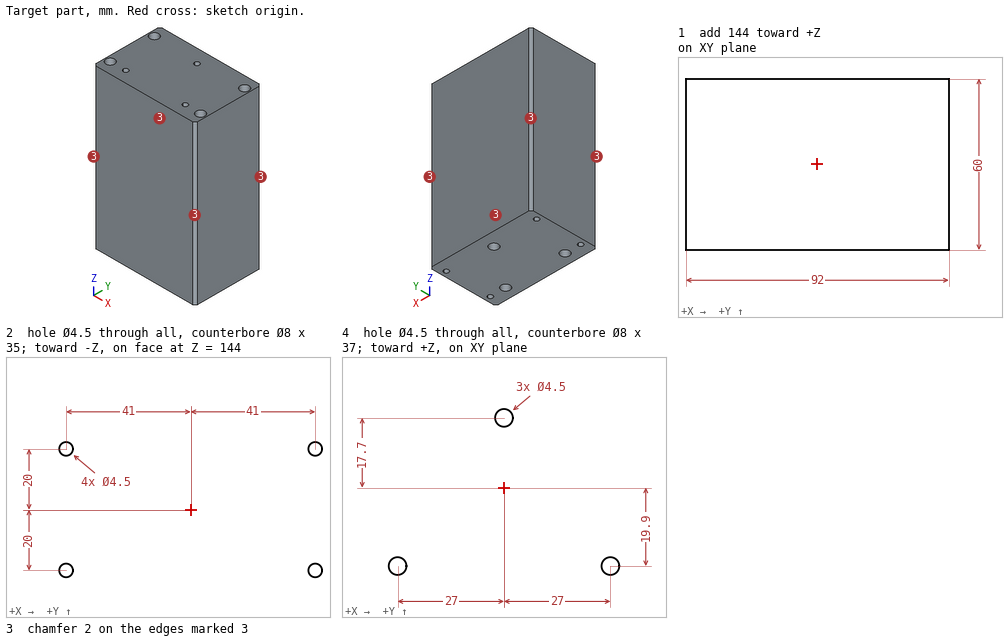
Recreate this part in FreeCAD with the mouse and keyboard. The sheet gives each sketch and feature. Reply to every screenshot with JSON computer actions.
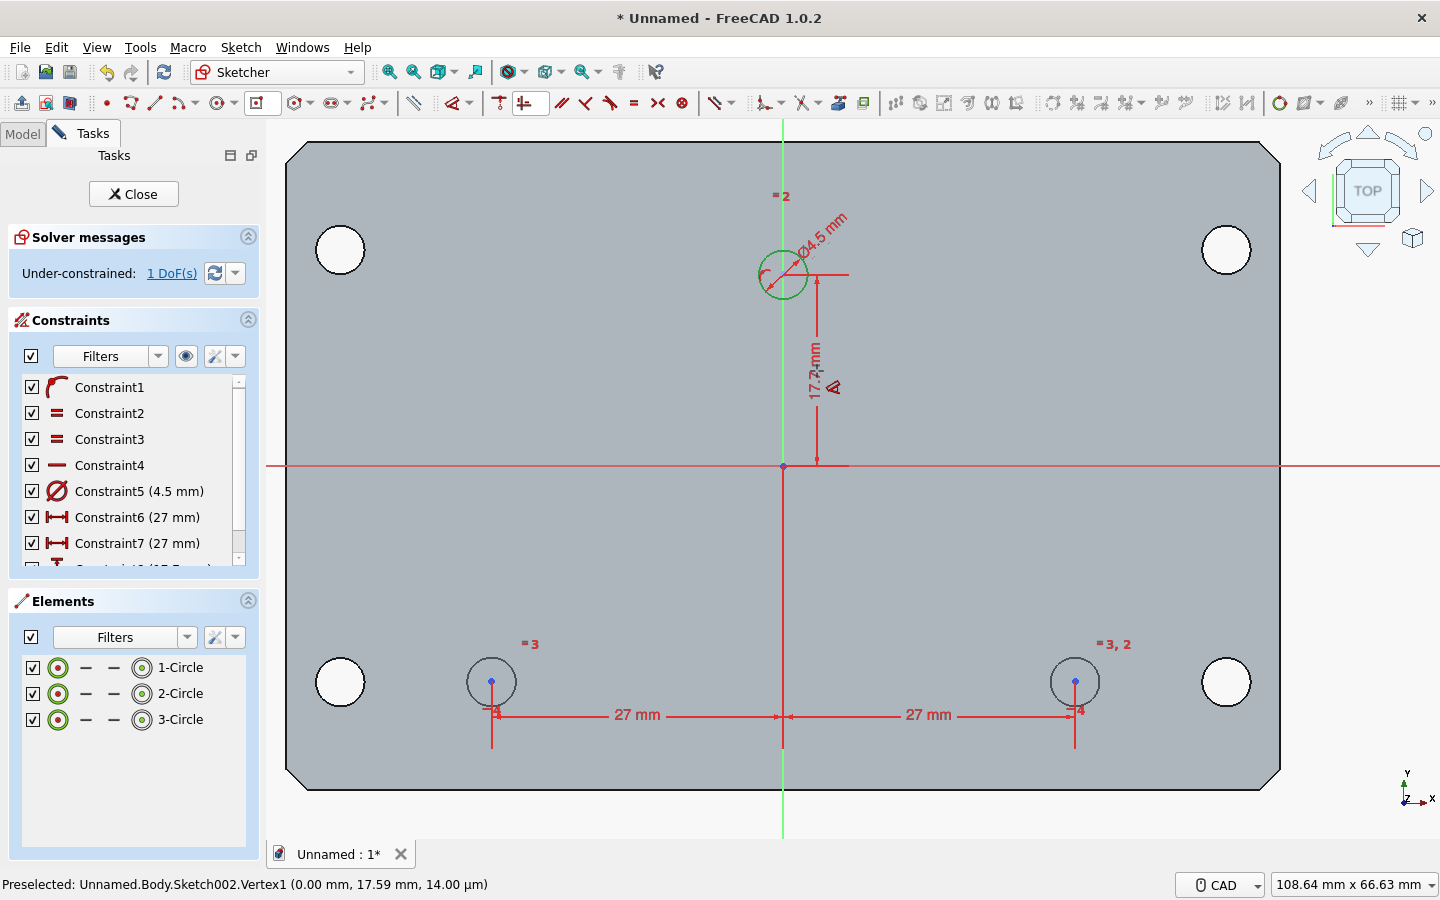
{"action": "left_click", "coordinate": [1075, 682]}
{"action": "left_click", "coordinate": [1109, 574]}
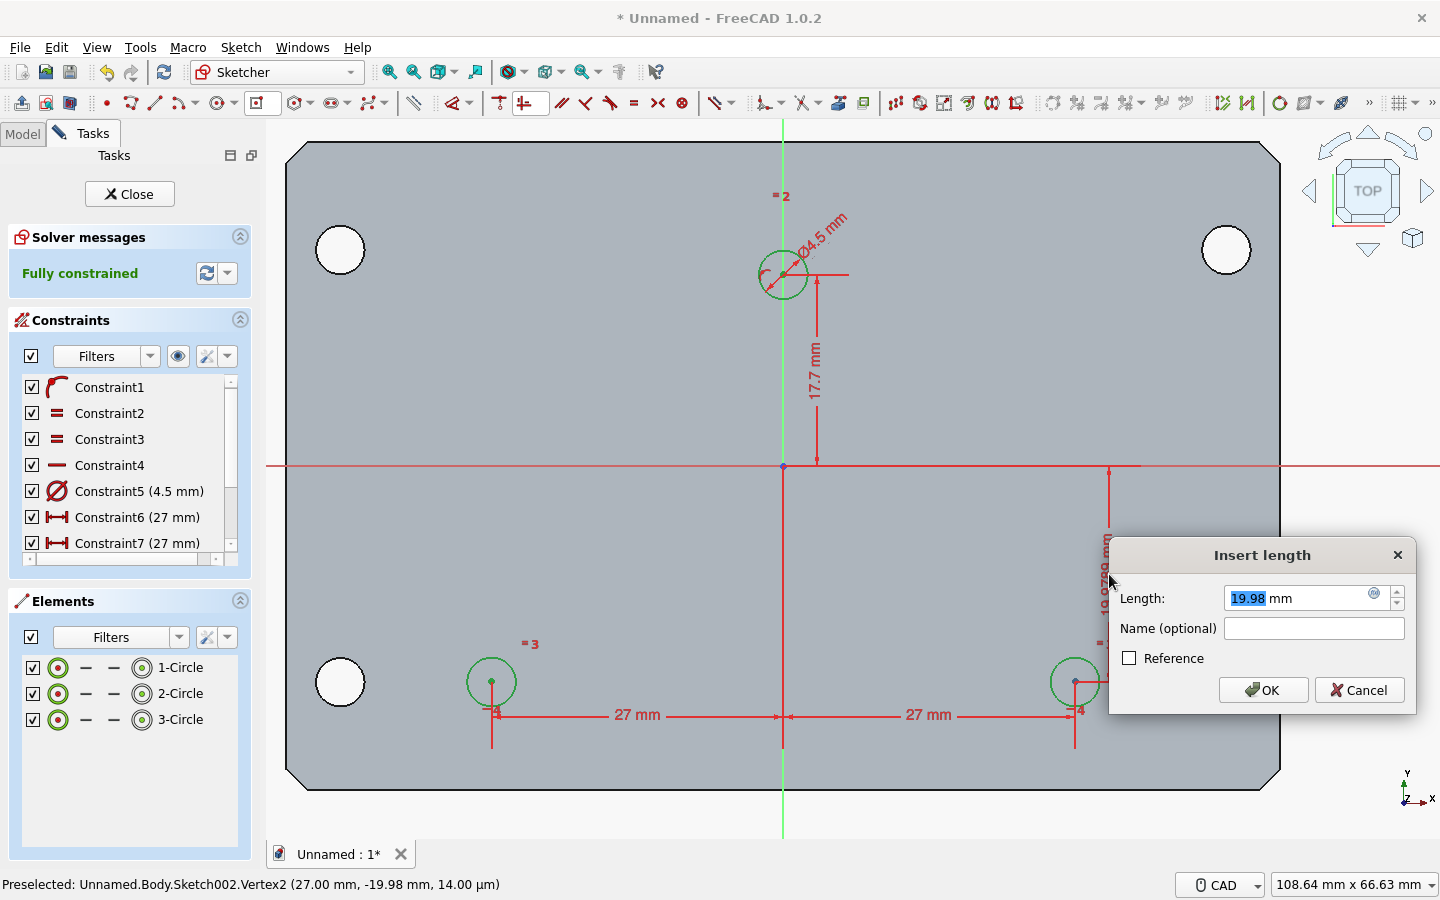
{"action": "type", "text": "19.9"}
{"action": "key", "text": "Return"}
{"action": "key", "text": "Escape"}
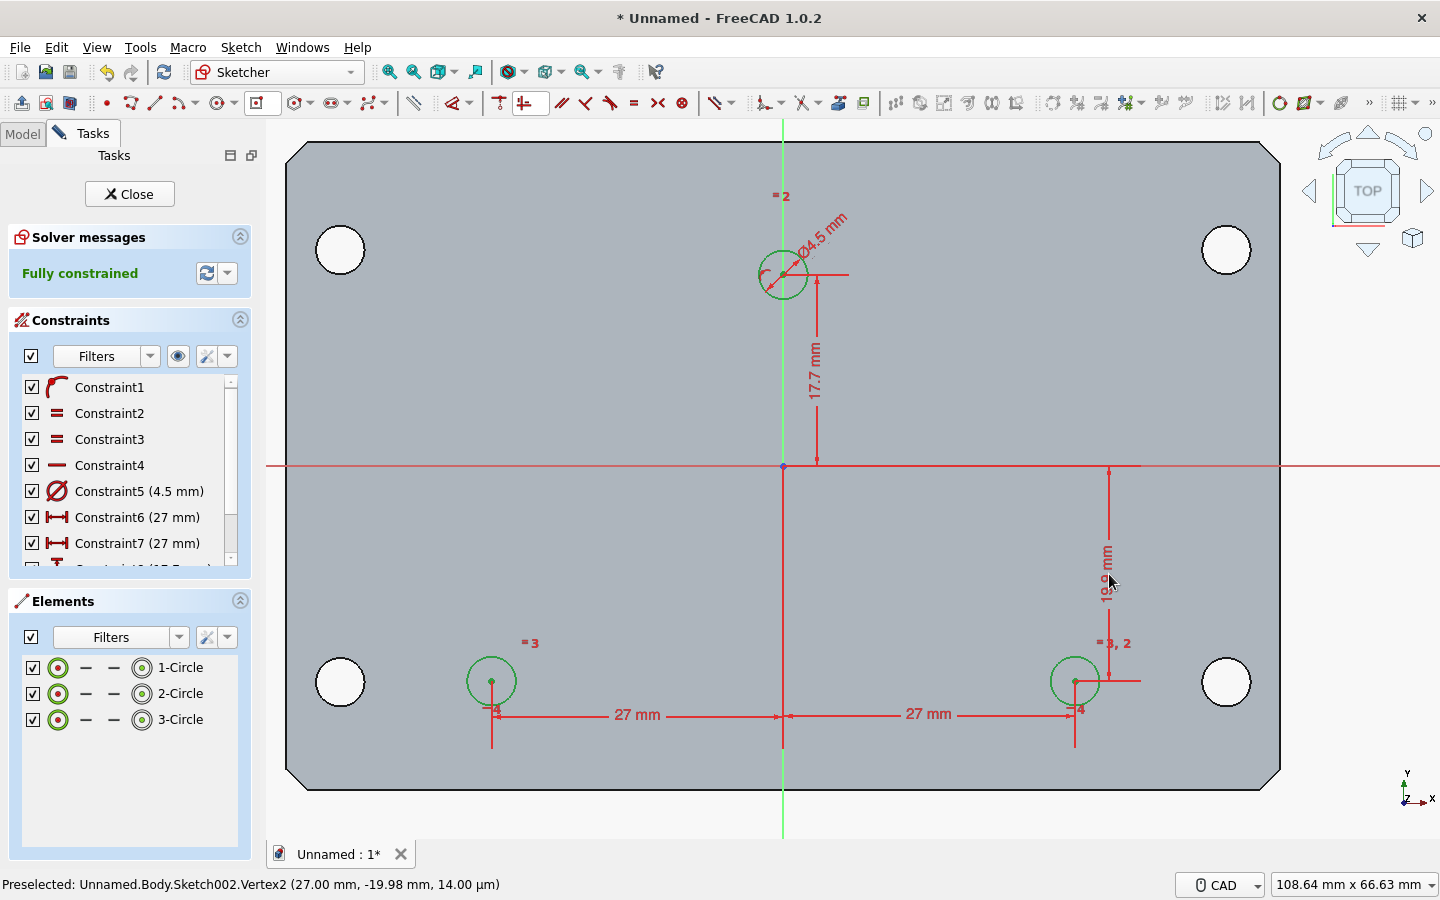
{"action": "left_click", "coordinate": [130, 194]}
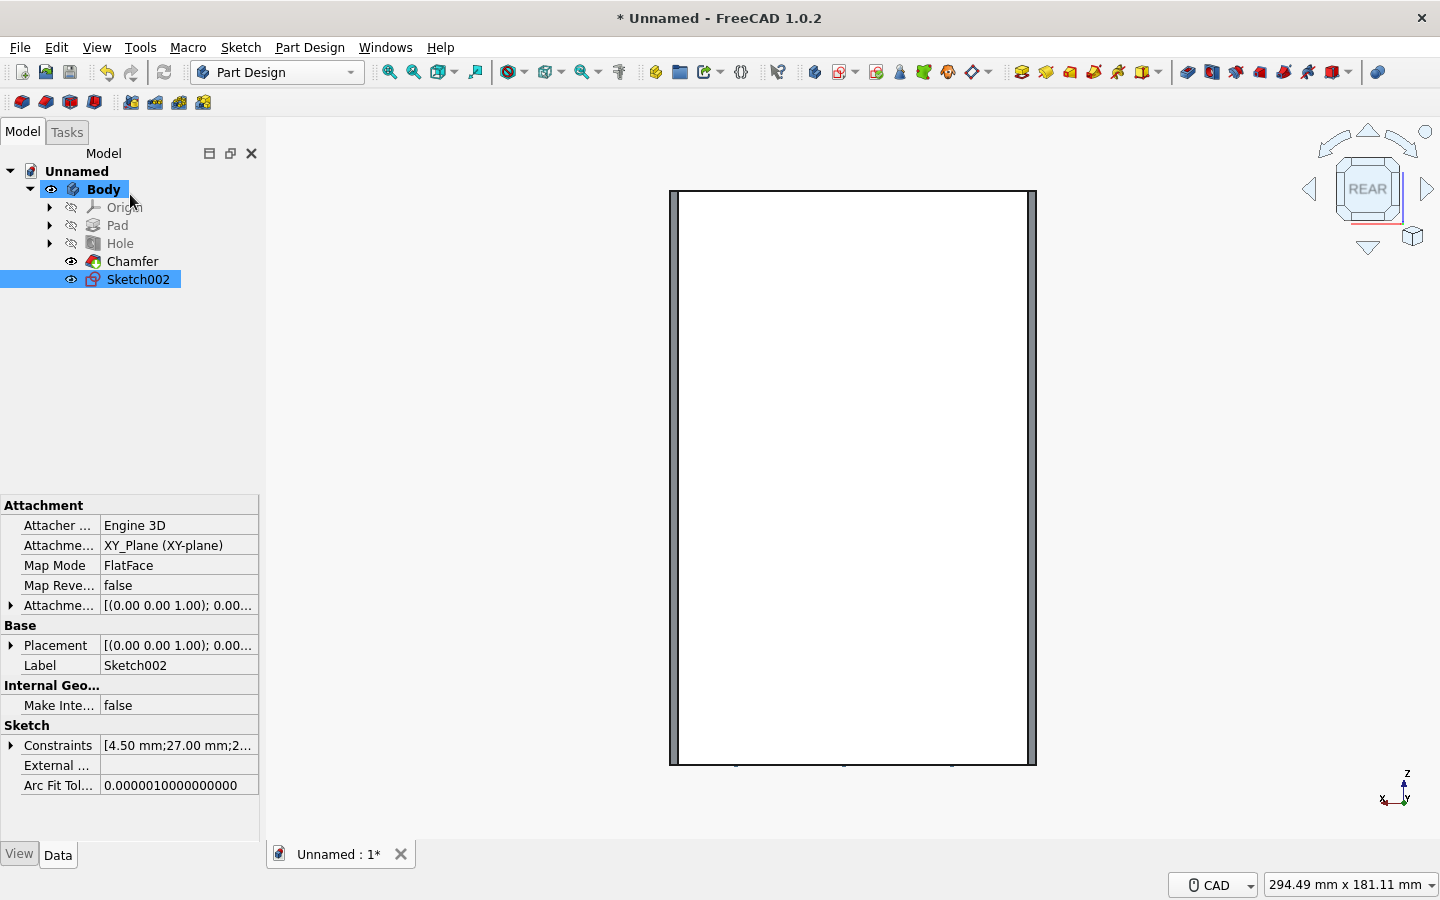
{"action": "left_click", "coordinate": [1212, 72]}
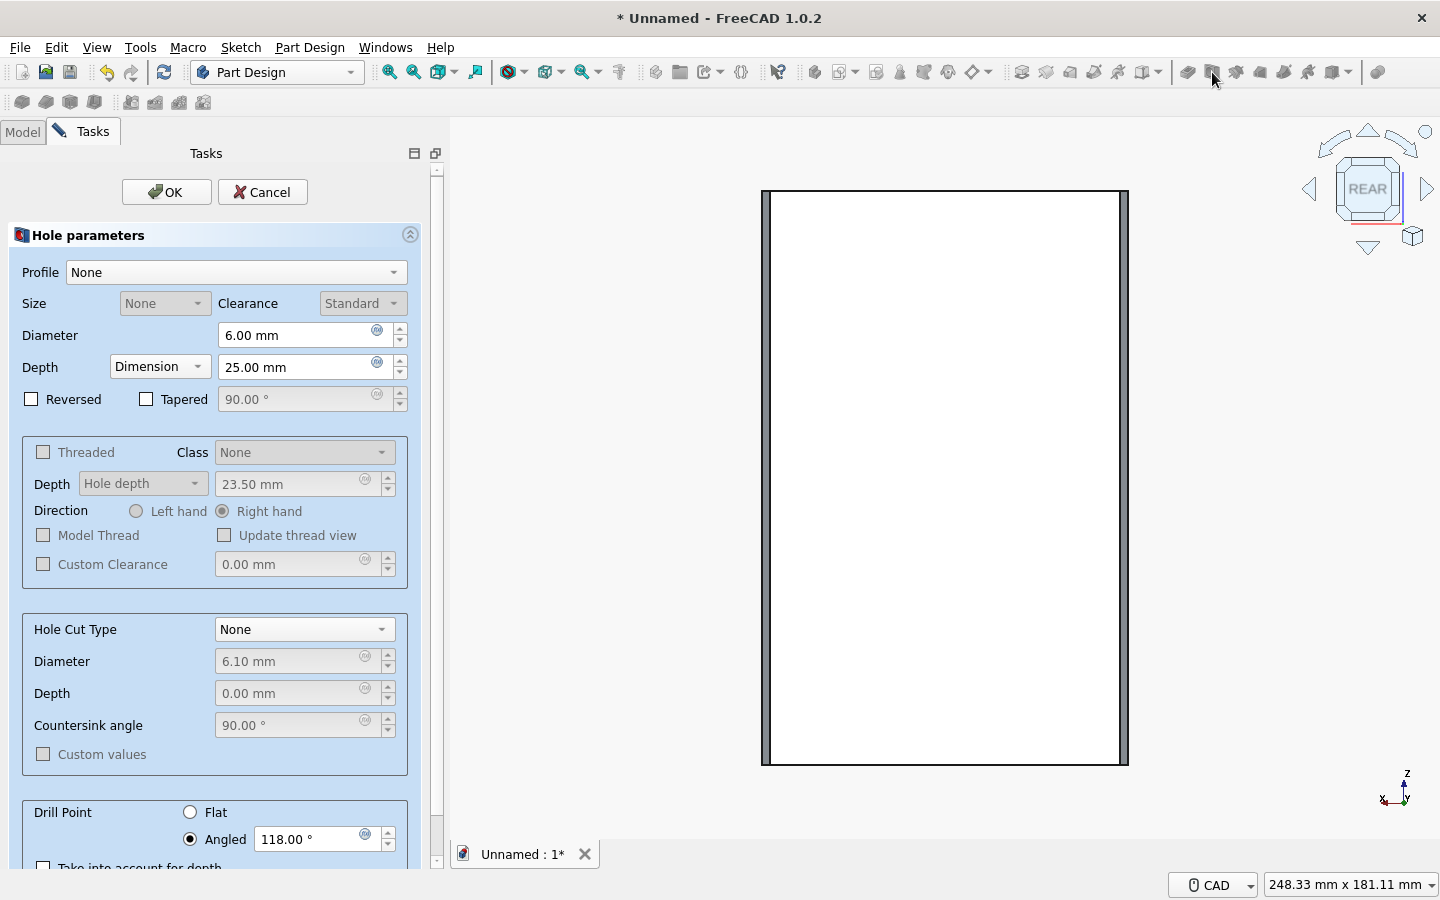
{"action": "triple_click", "coordinate": [305, 335]}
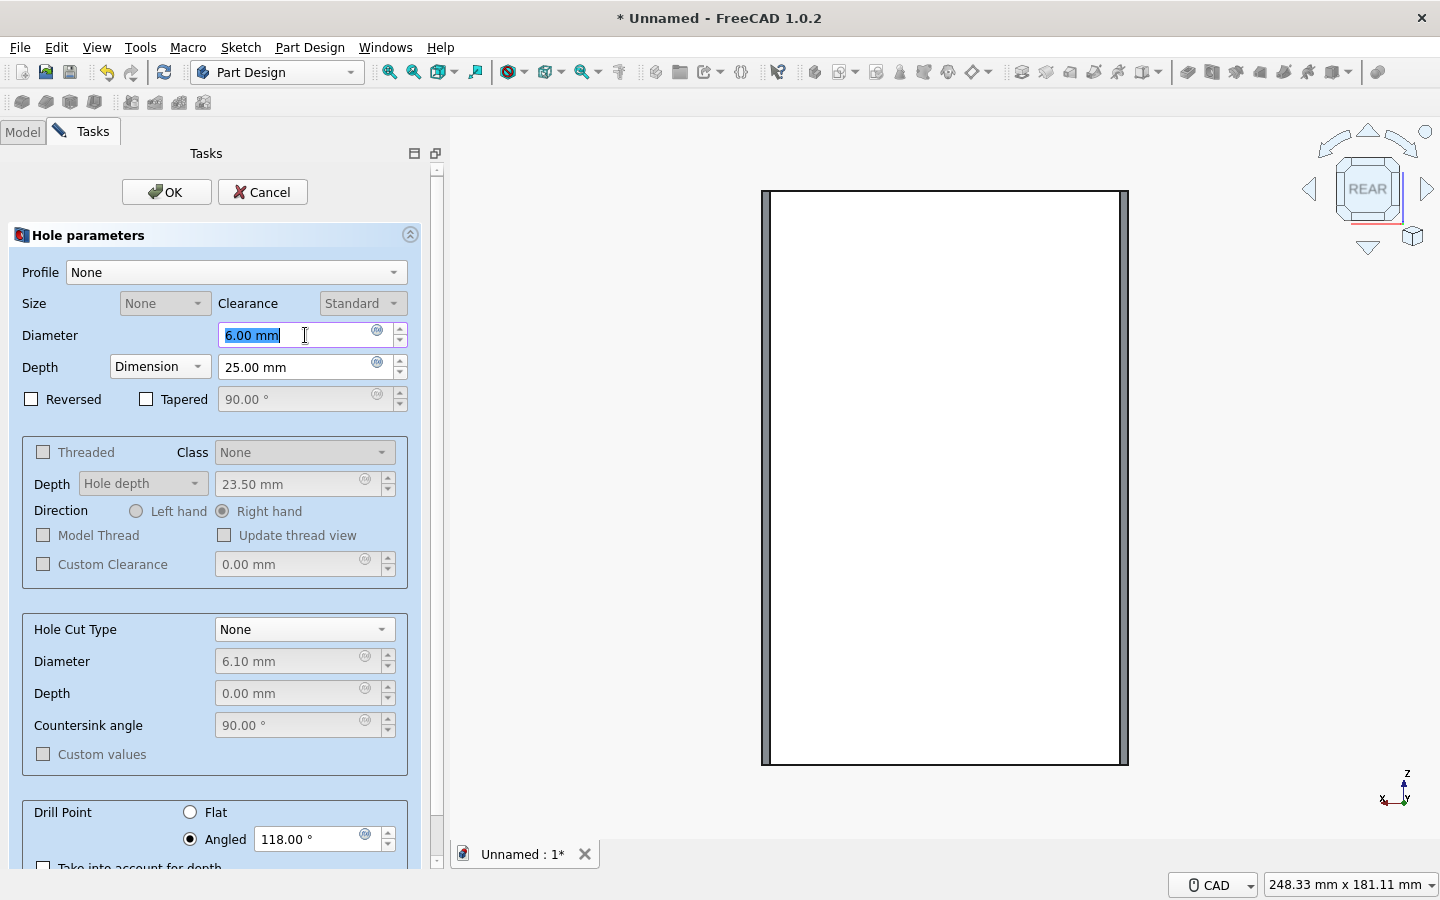
{"action": "type", "text": "4.5"}
{"action": "key", "text": "Tab"}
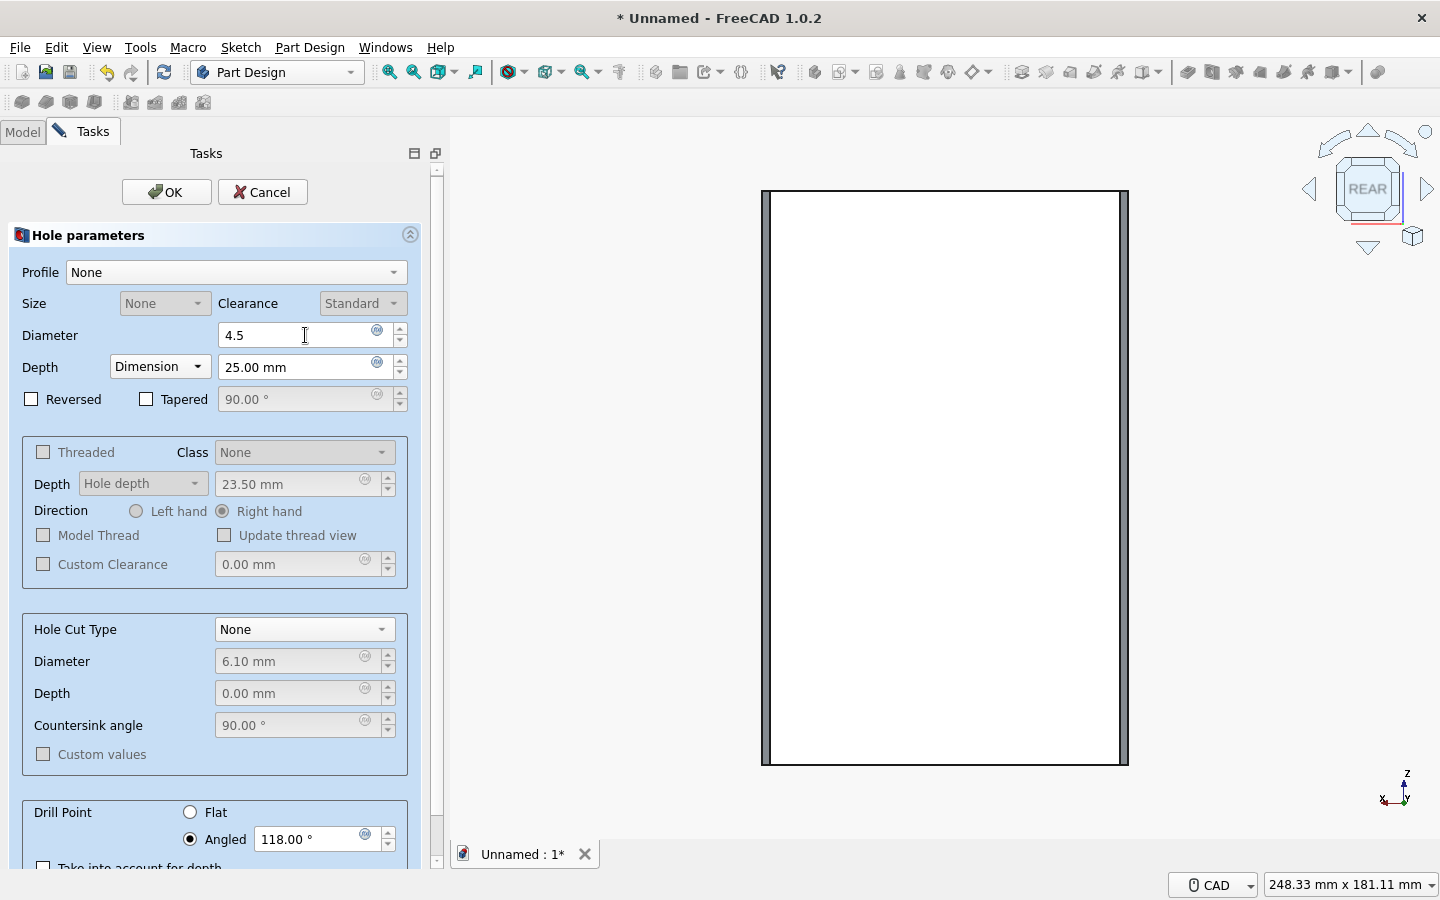
{"action": "left_click", "coordinate": [161, 366]}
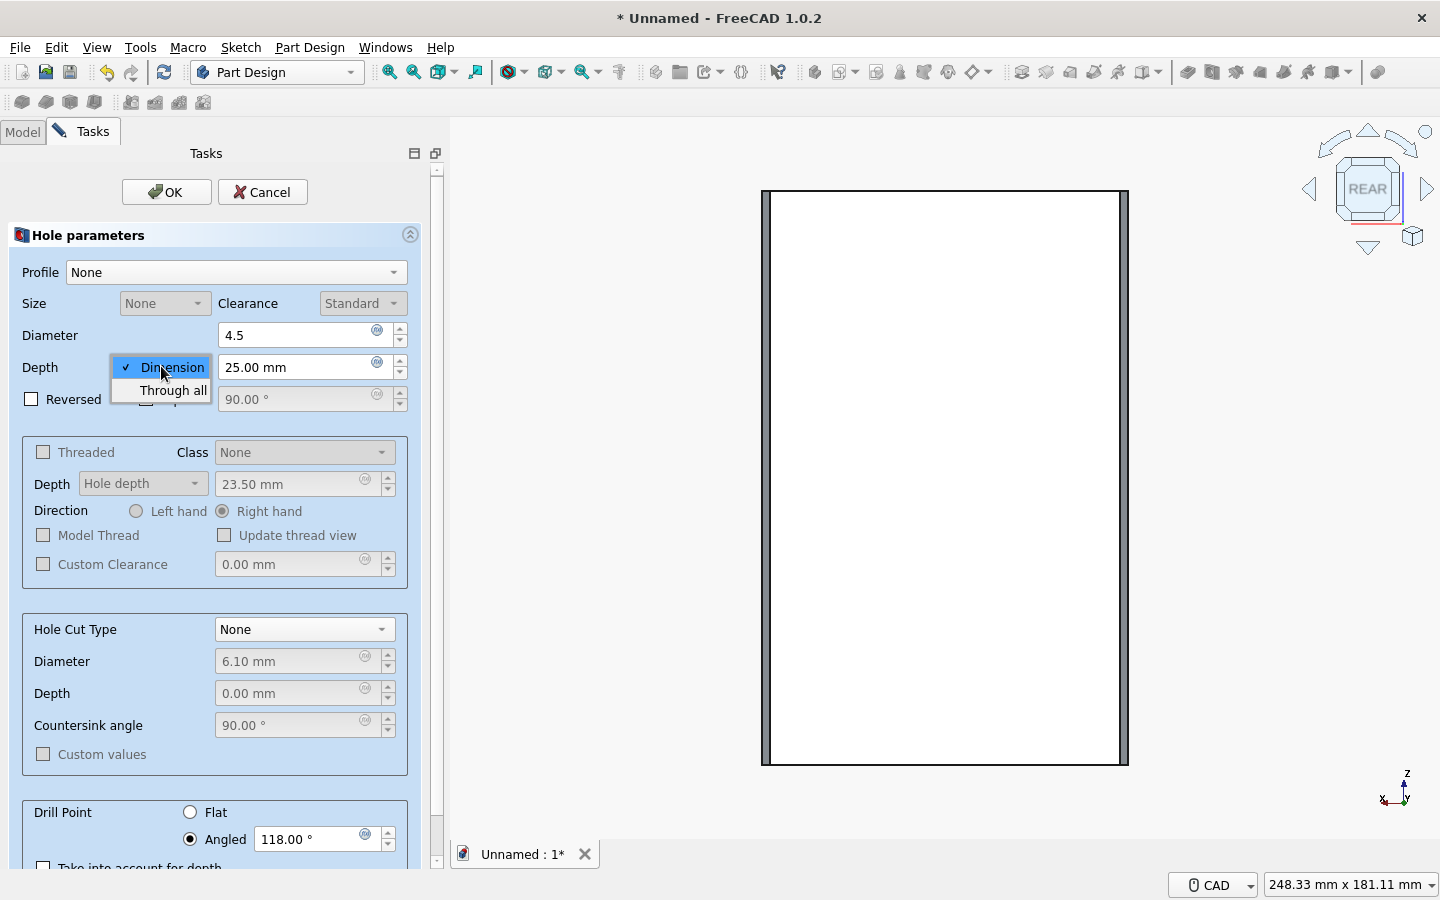
{"action": "left_click", "coordinate": [160, 390]}